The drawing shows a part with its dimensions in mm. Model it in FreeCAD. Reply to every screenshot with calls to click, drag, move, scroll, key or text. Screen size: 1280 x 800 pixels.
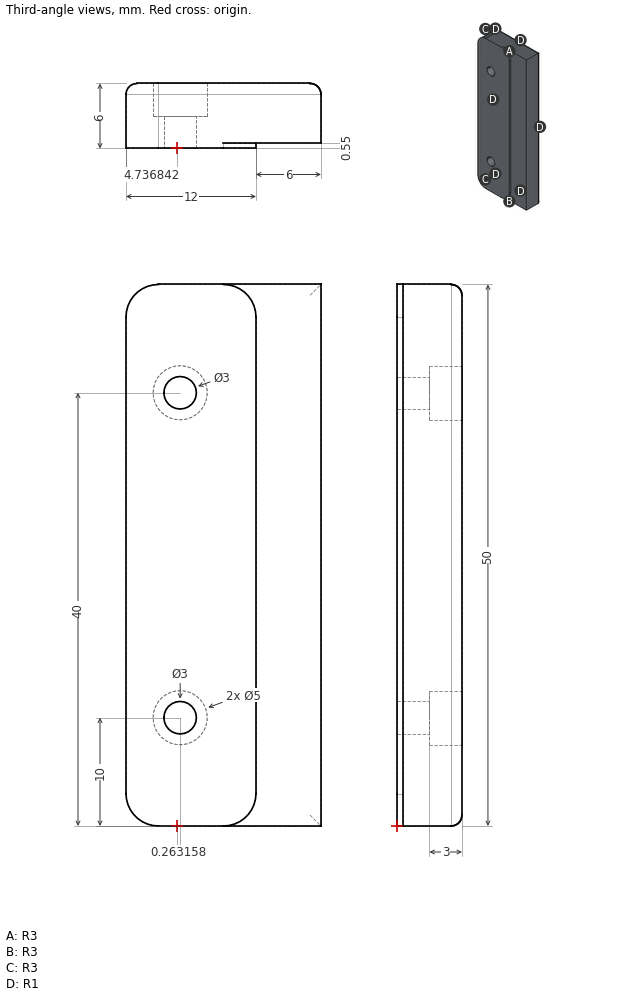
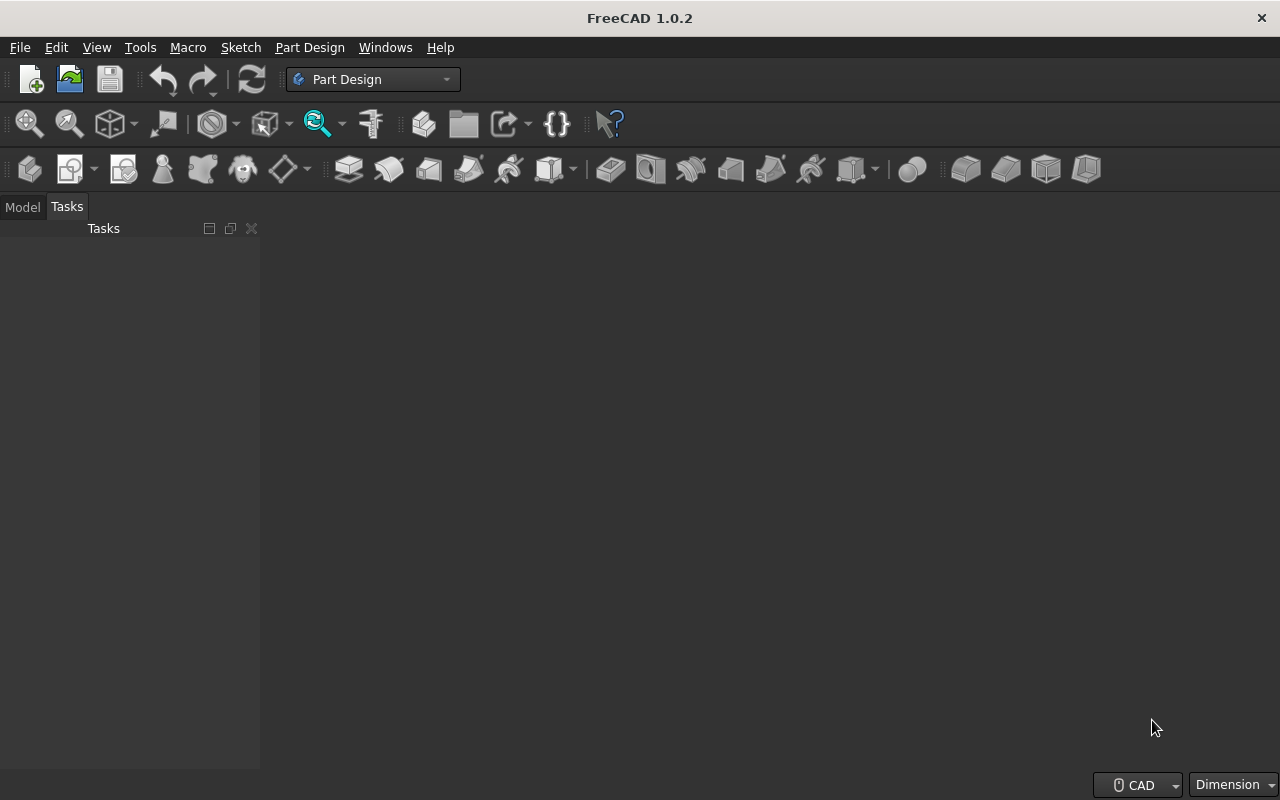
click(30, 80)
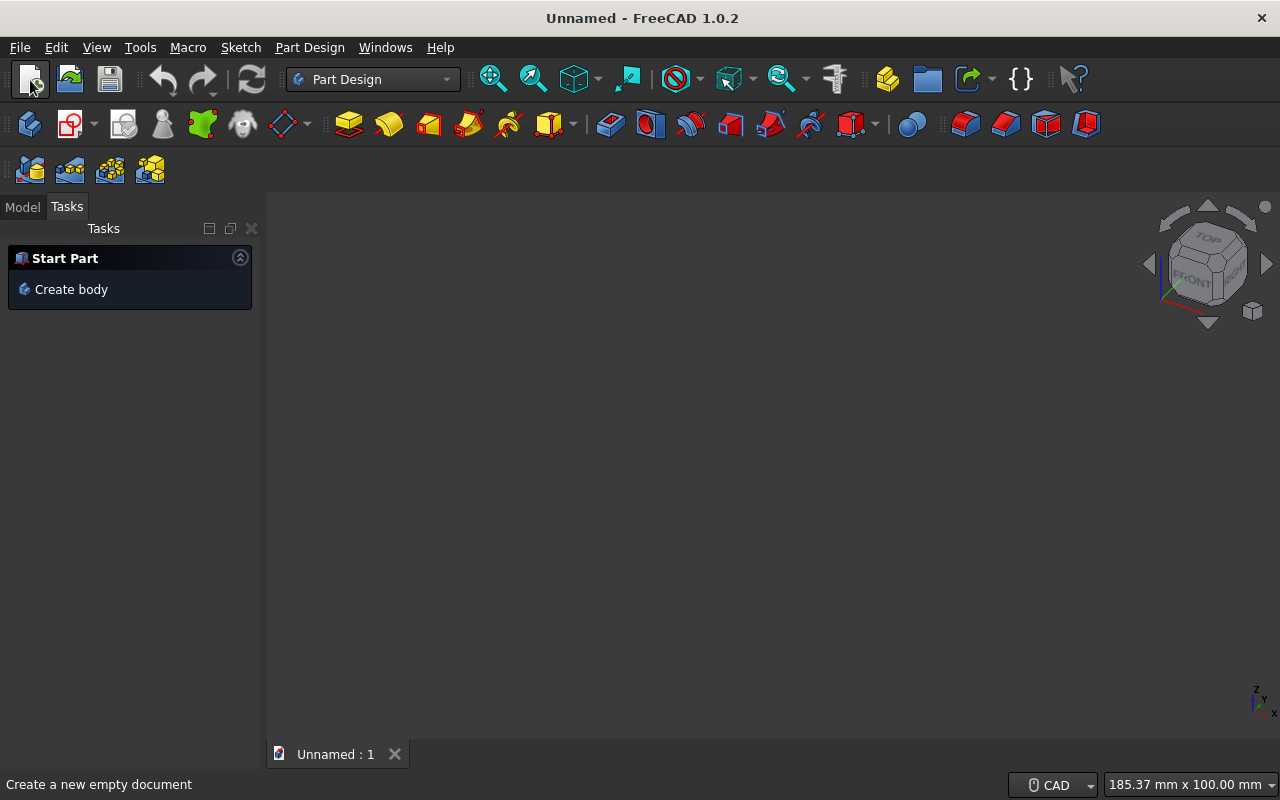
click(70, 124)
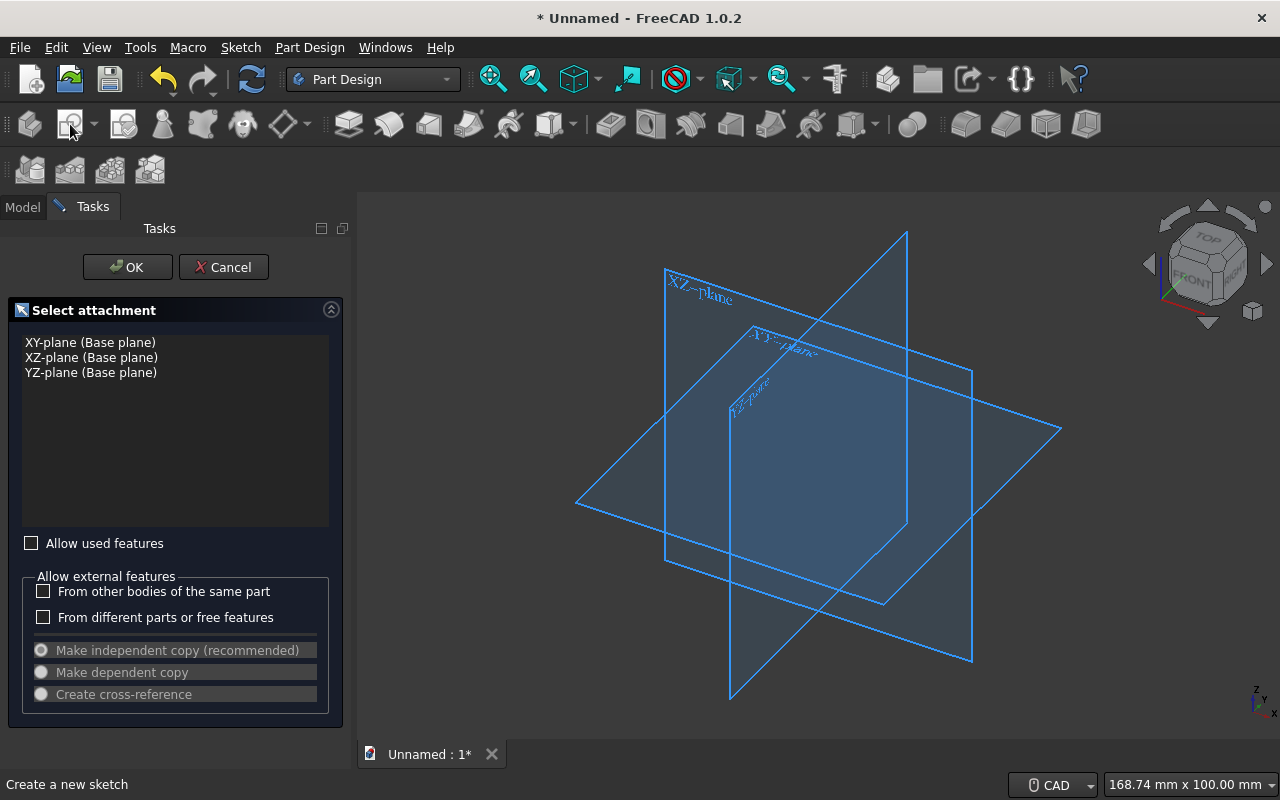
click(82, 342)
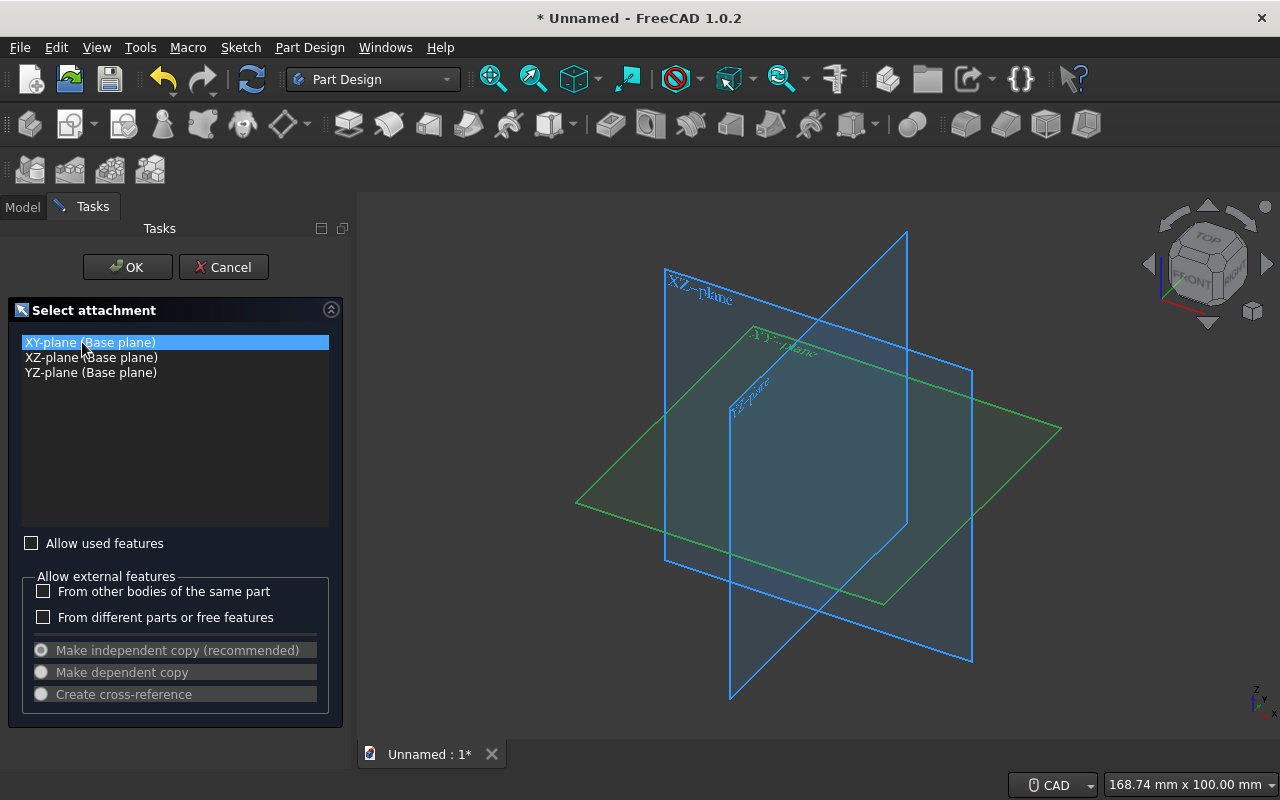
click(128, 267)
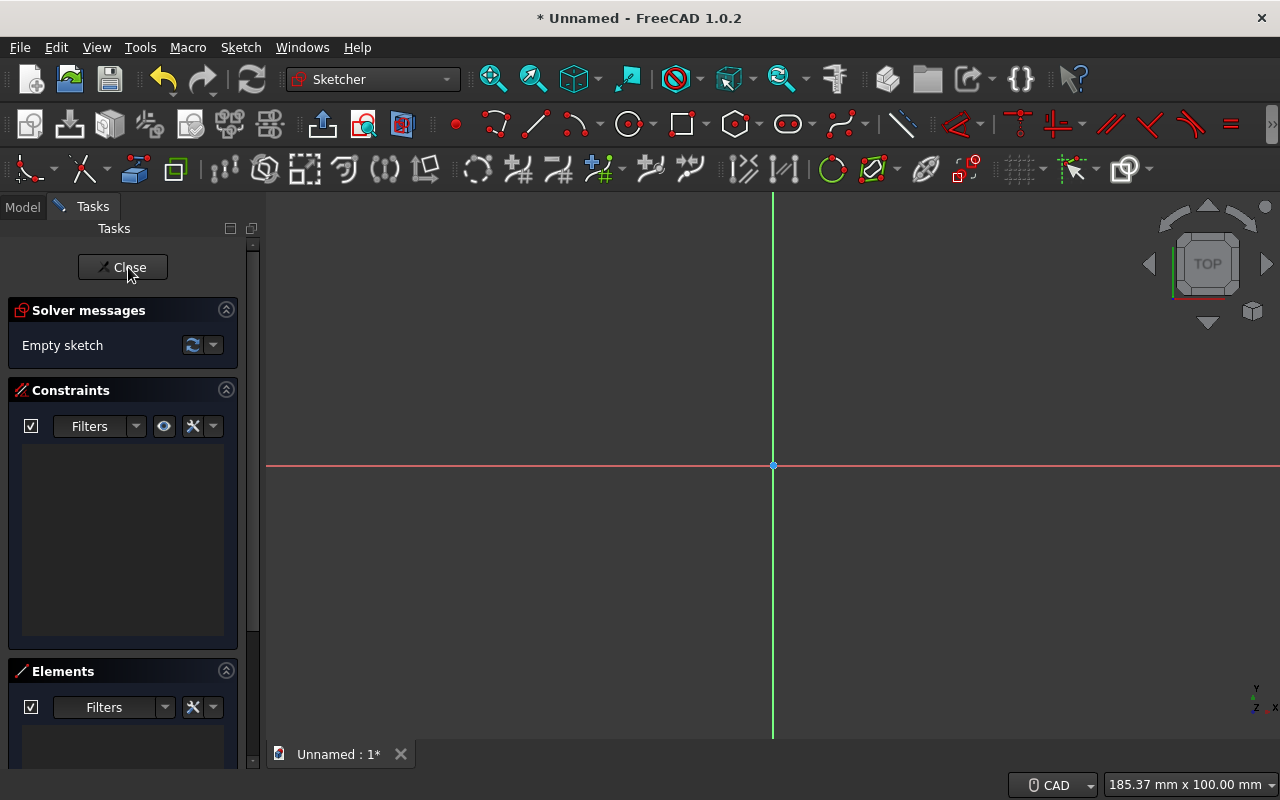
scroll(815, 446, up, 9)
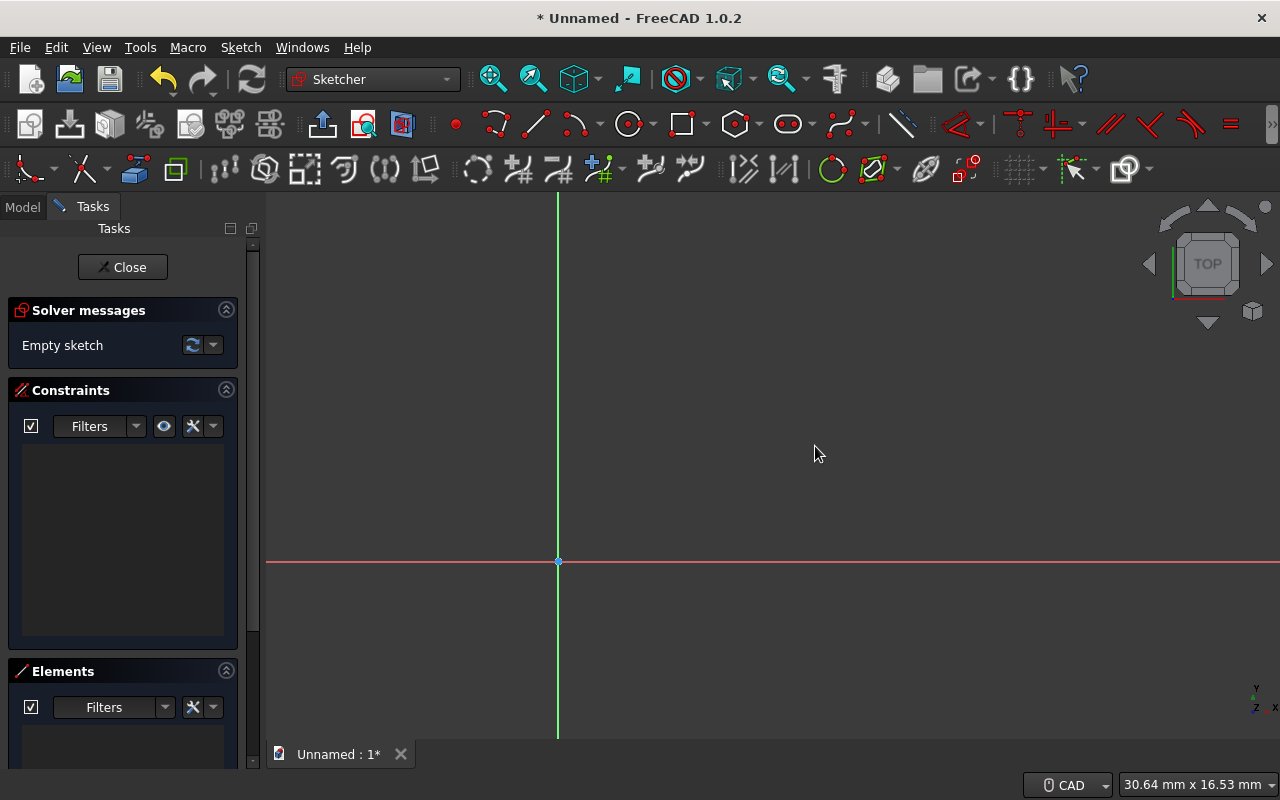
click(496, 124)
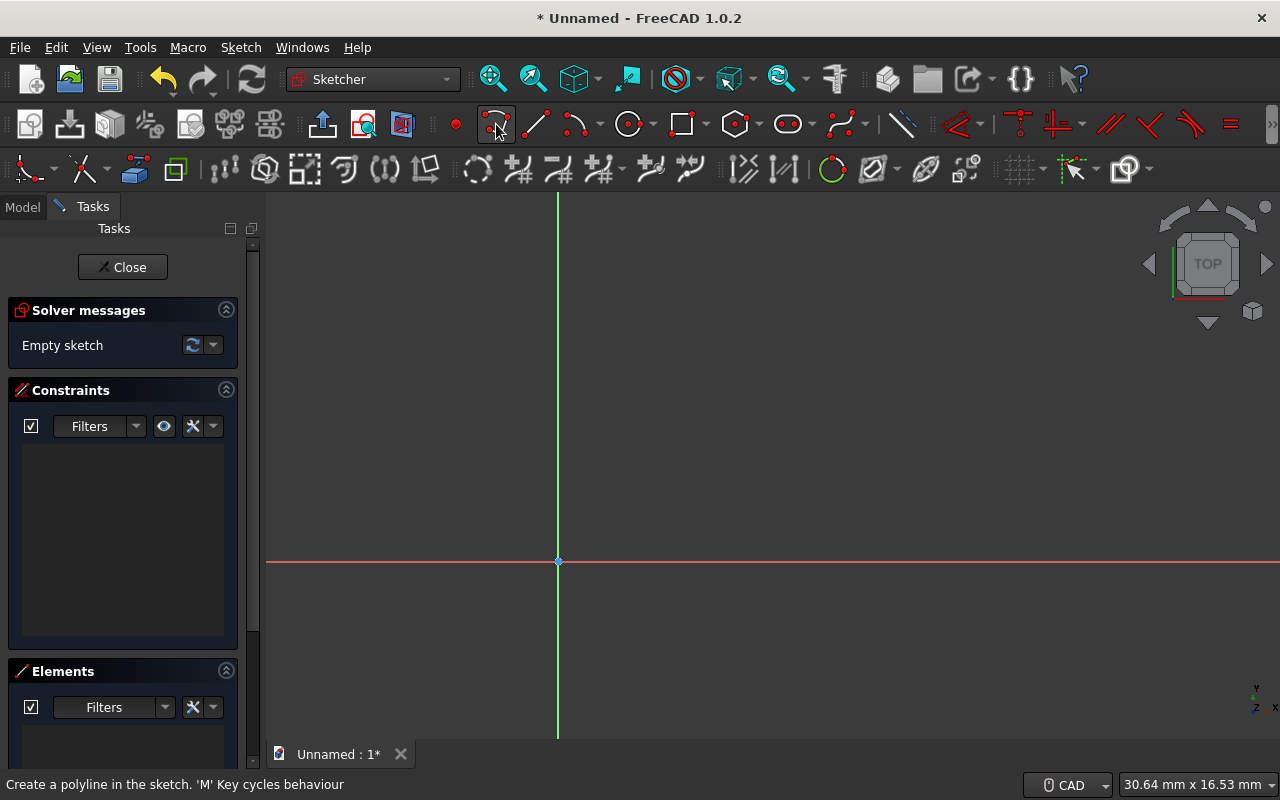
click(401, 562)
click(799, 553)
click(799, 543)
click(997, 543)
click(997, 363)
click(401, 363)
click(401, 562)
key(Escape)
key(Escape)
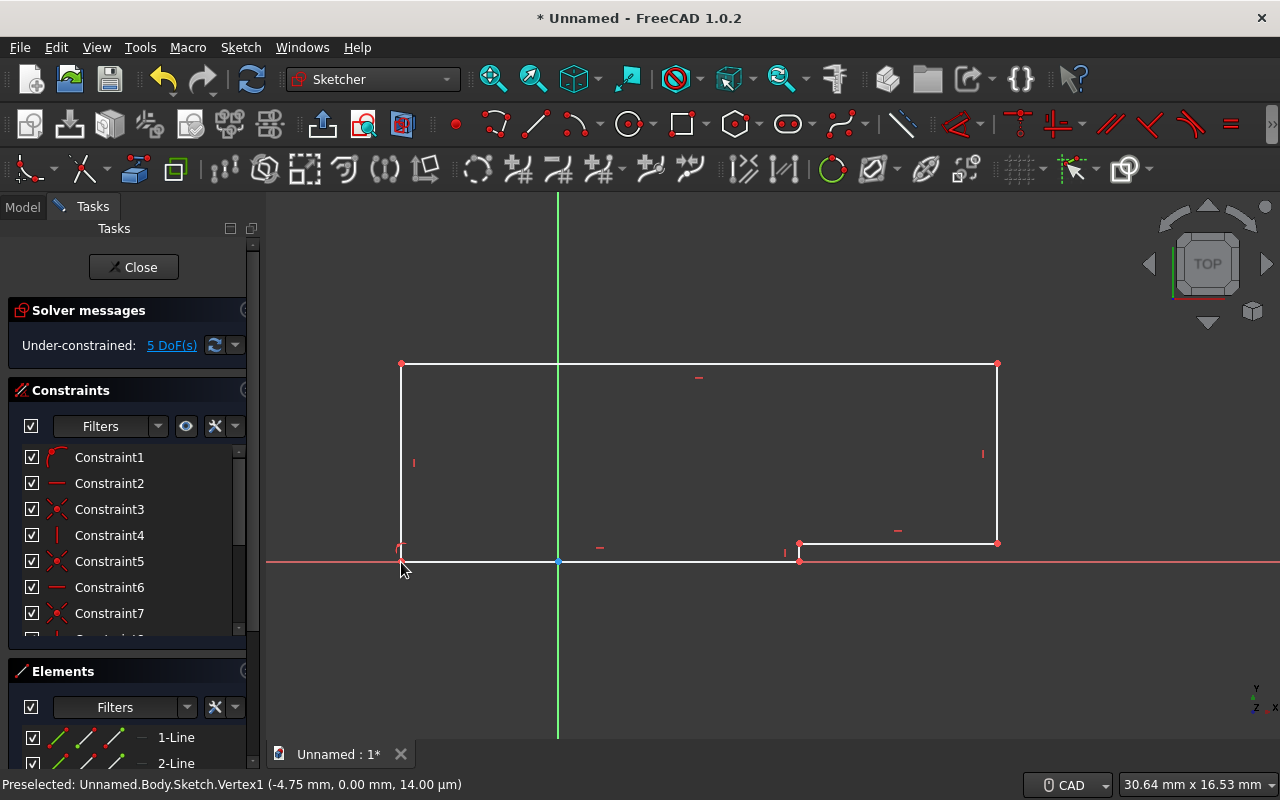
key(d)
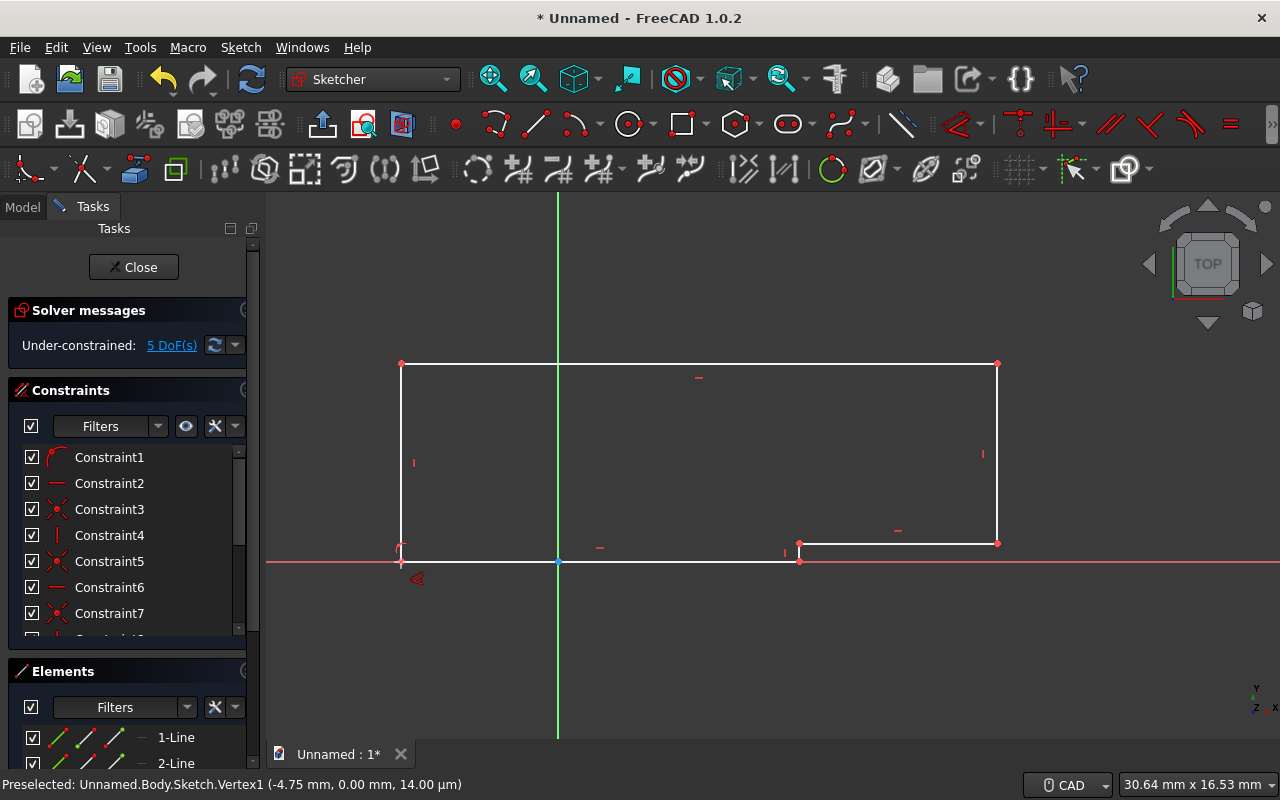
click(858, 544)
click(898, 578)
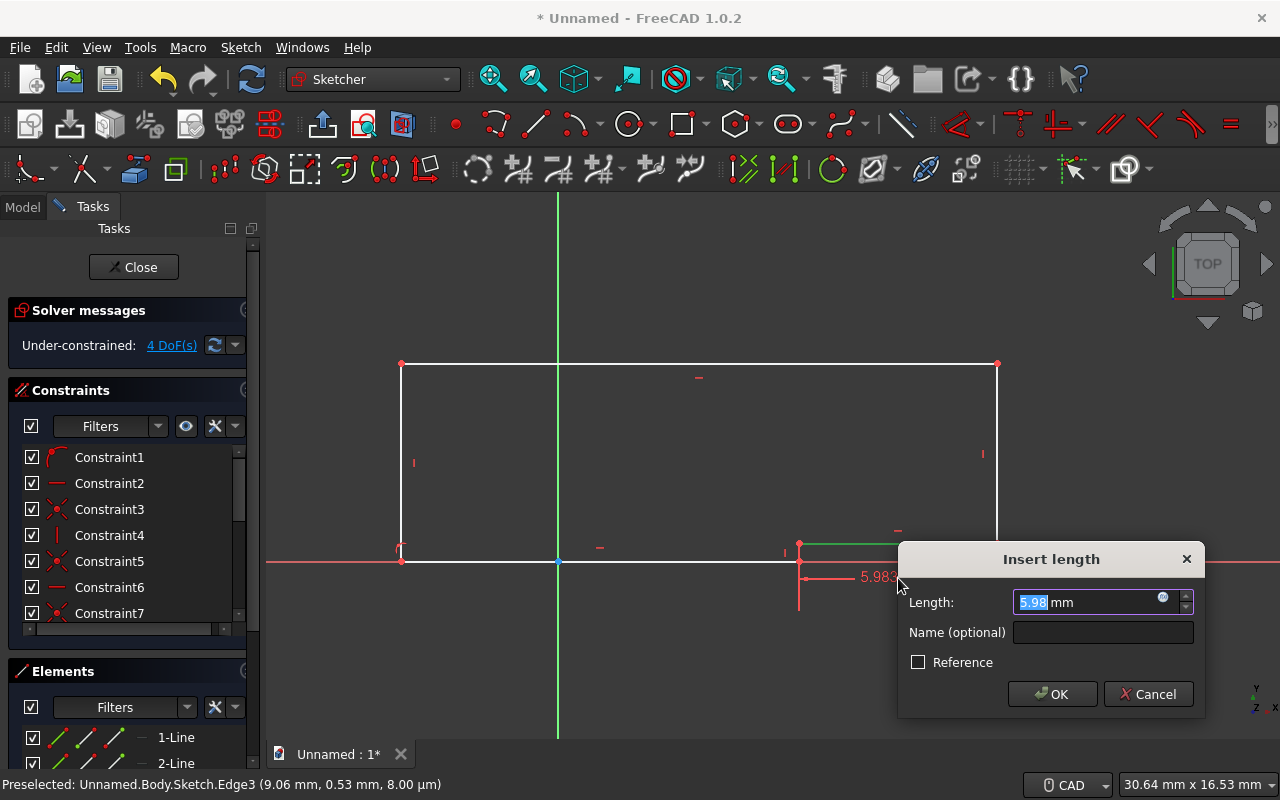
text(6)
key(Return)